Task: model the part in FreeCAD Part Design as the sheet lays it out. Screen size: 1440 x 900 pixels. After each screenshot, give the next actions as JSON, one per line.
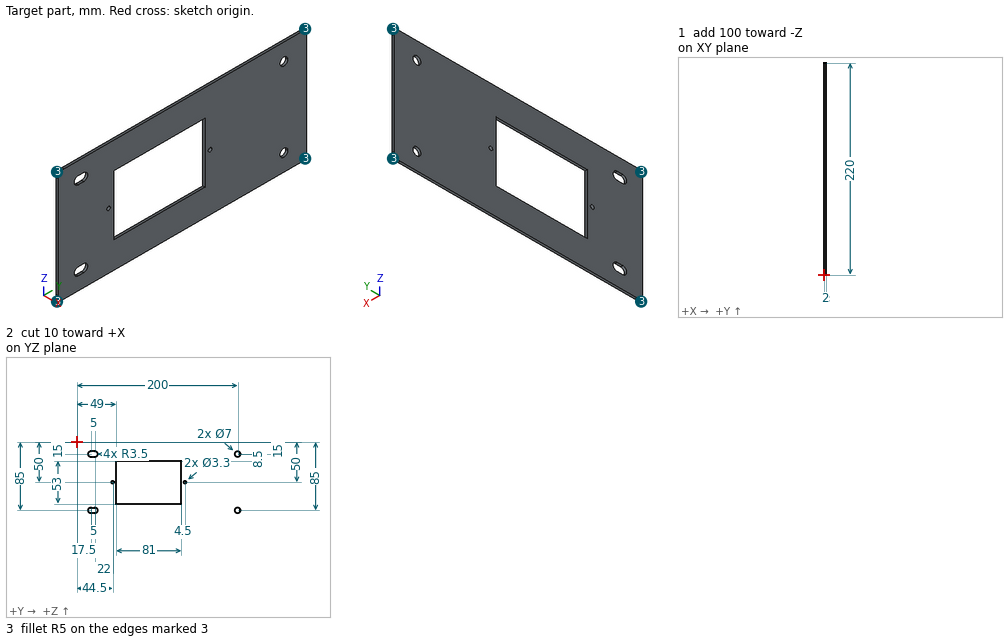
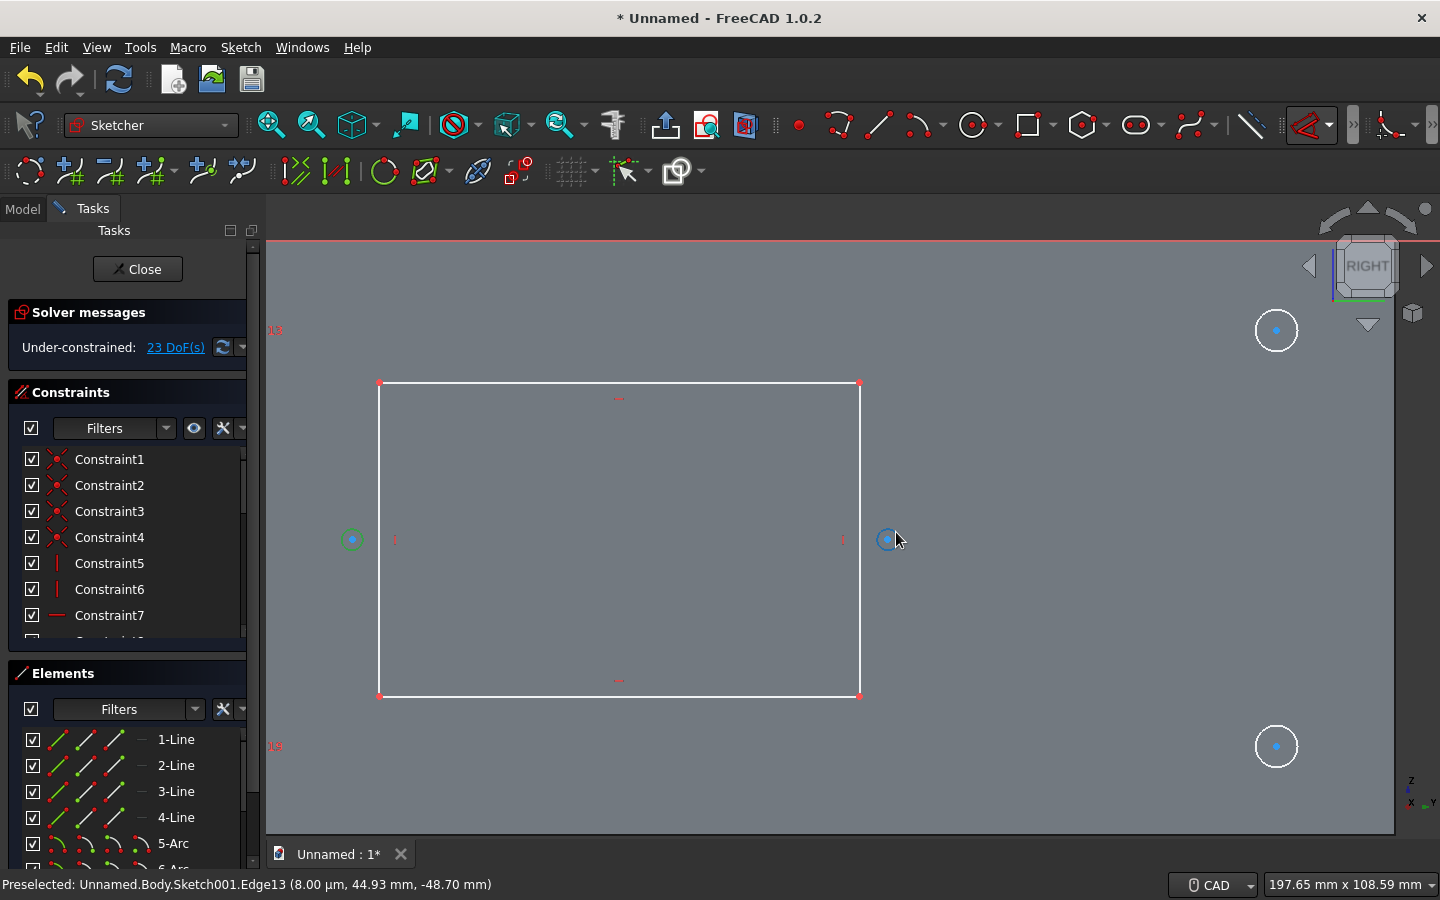
{"action": "left_click", "coordinate": [895, 532]}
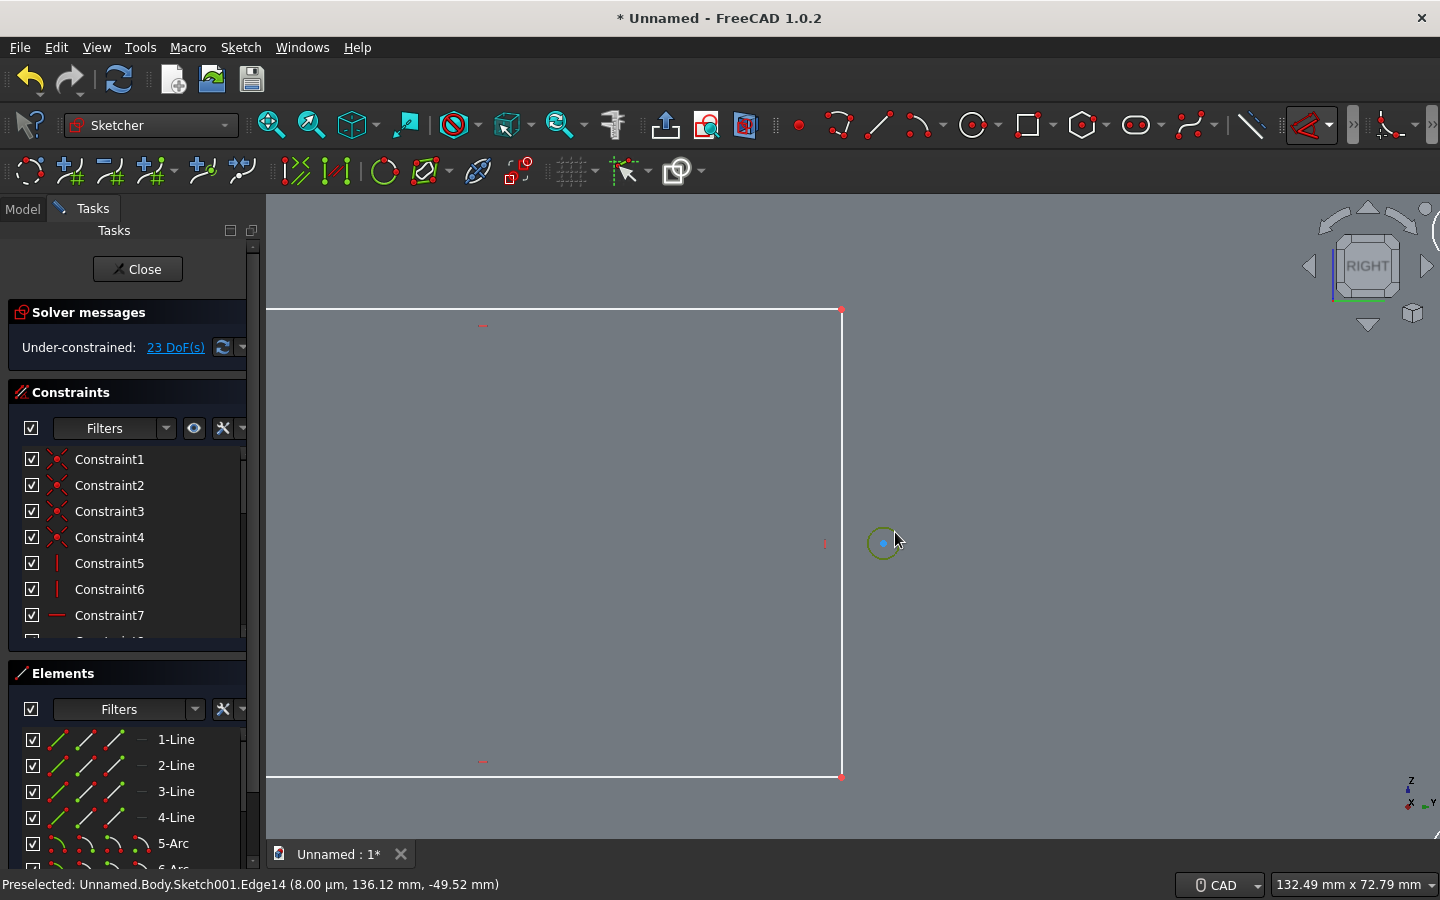
{"action": "key", "text": "e"}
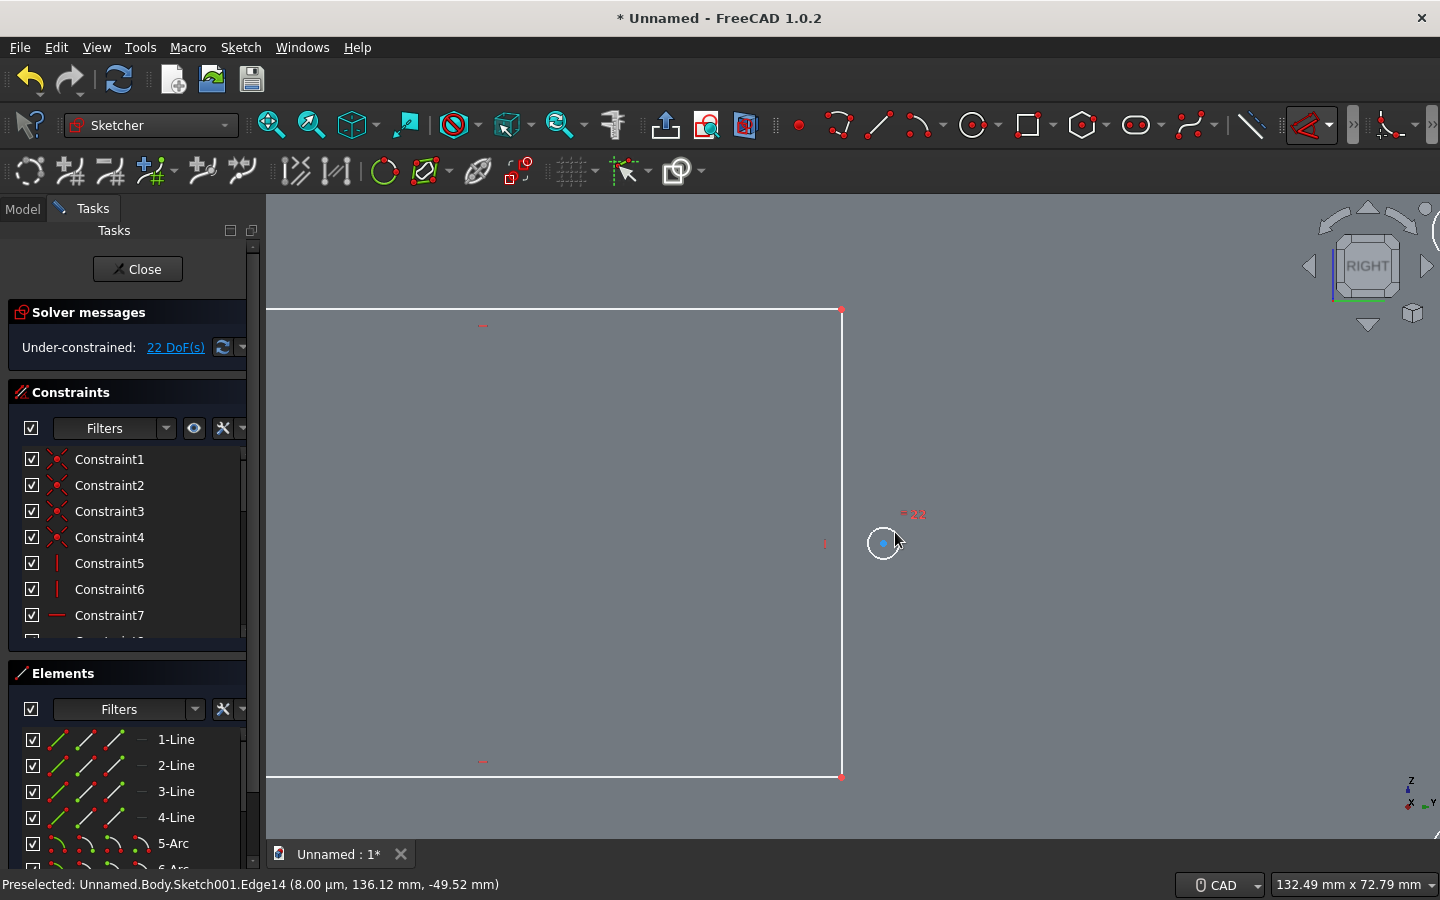
{"action": "scroll", "coordinate": [896, 532], "scroll_direction": "down", "scroll_amount": 5}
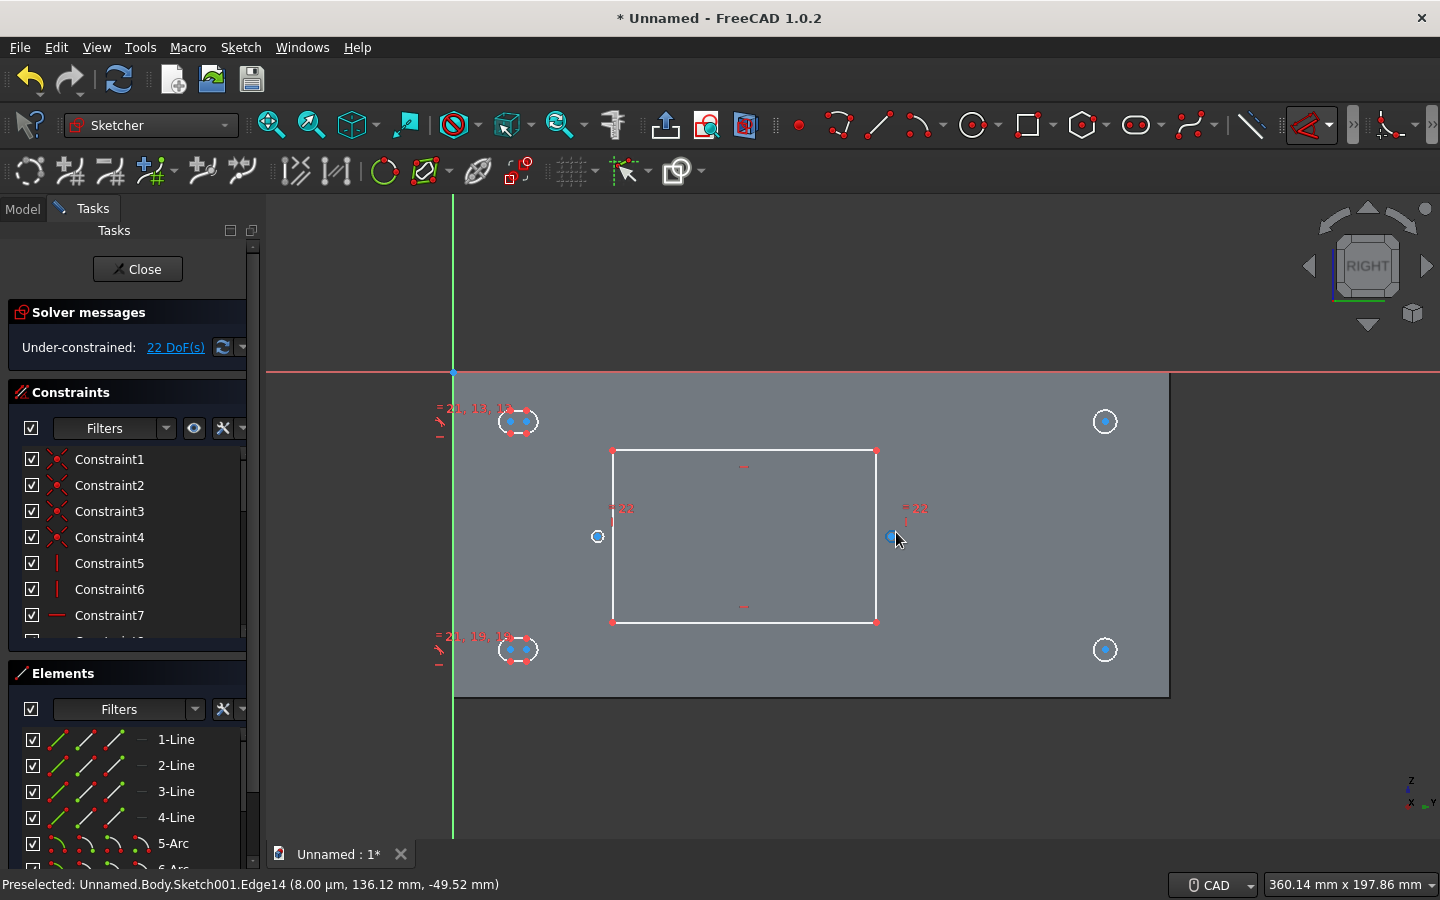
{"action": "left_click", "coordinate": [1113, 414]}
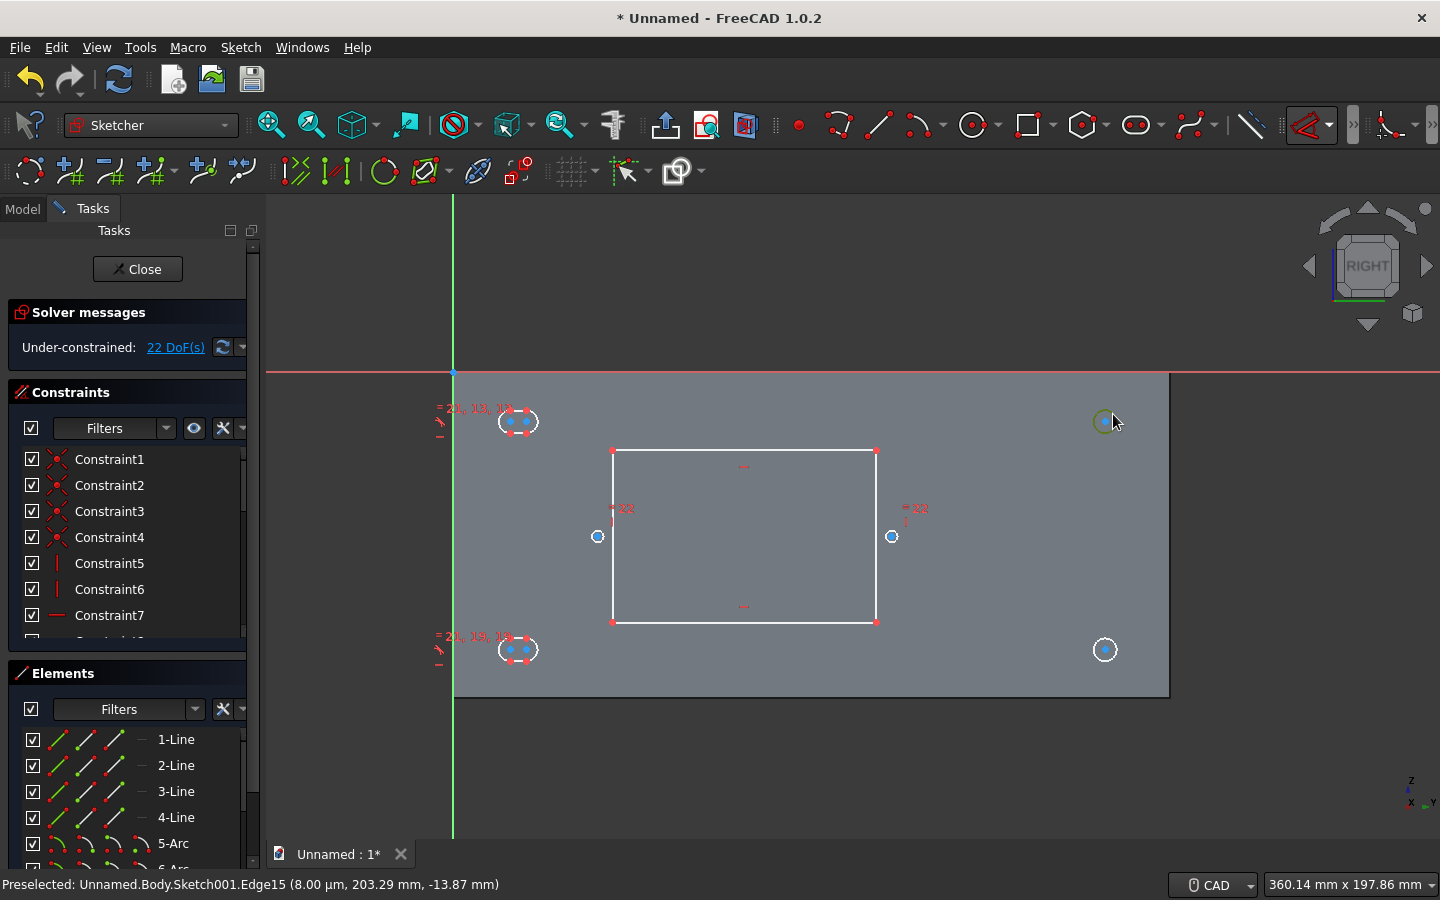
{"action": "left_click", "coordinate": [1113, 642]}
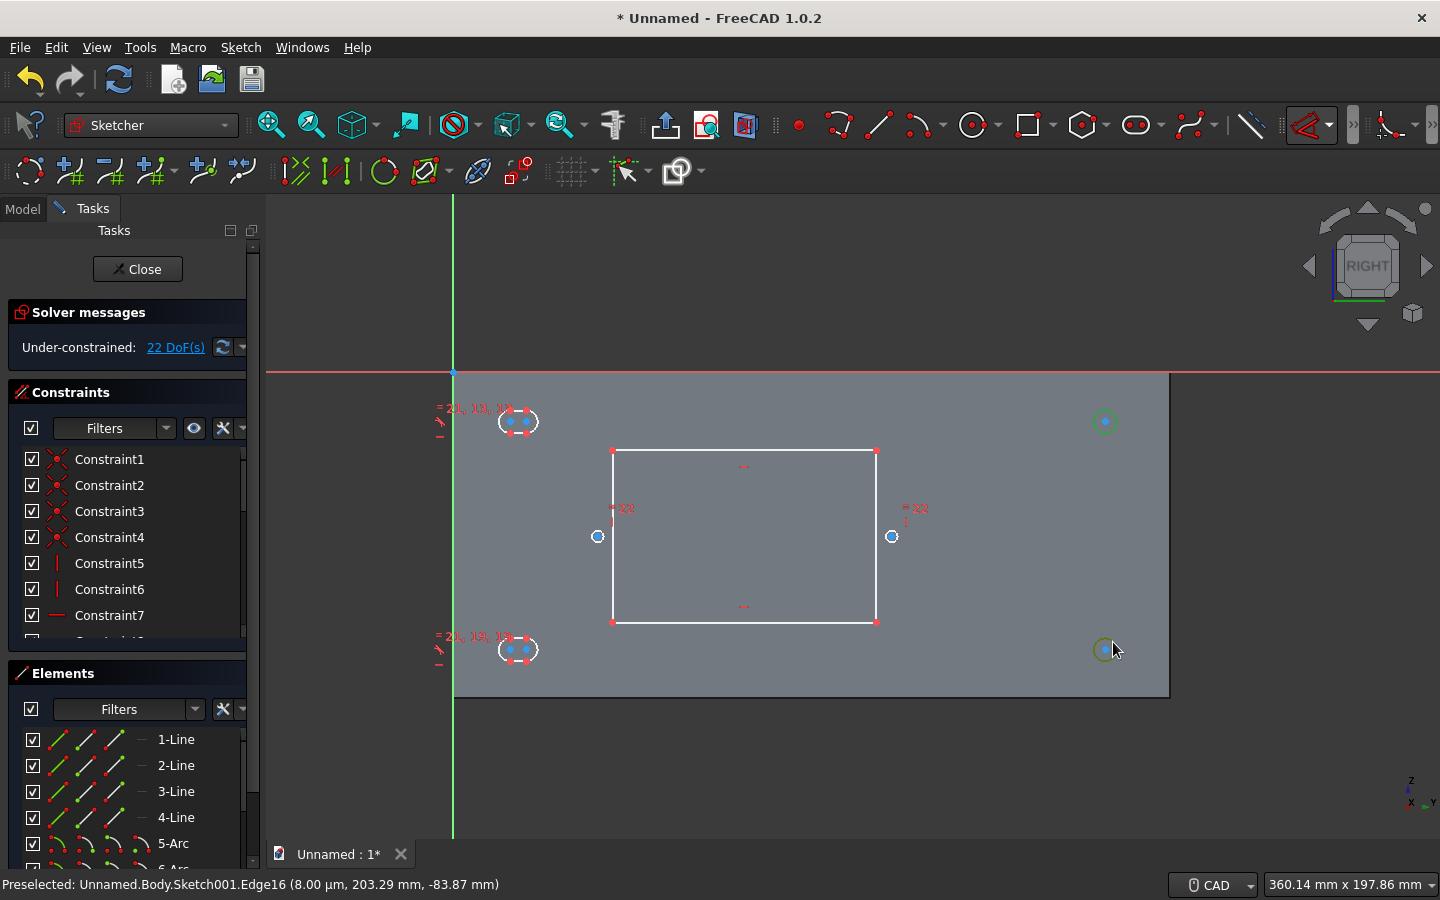
{"action": "key", "text": "e"}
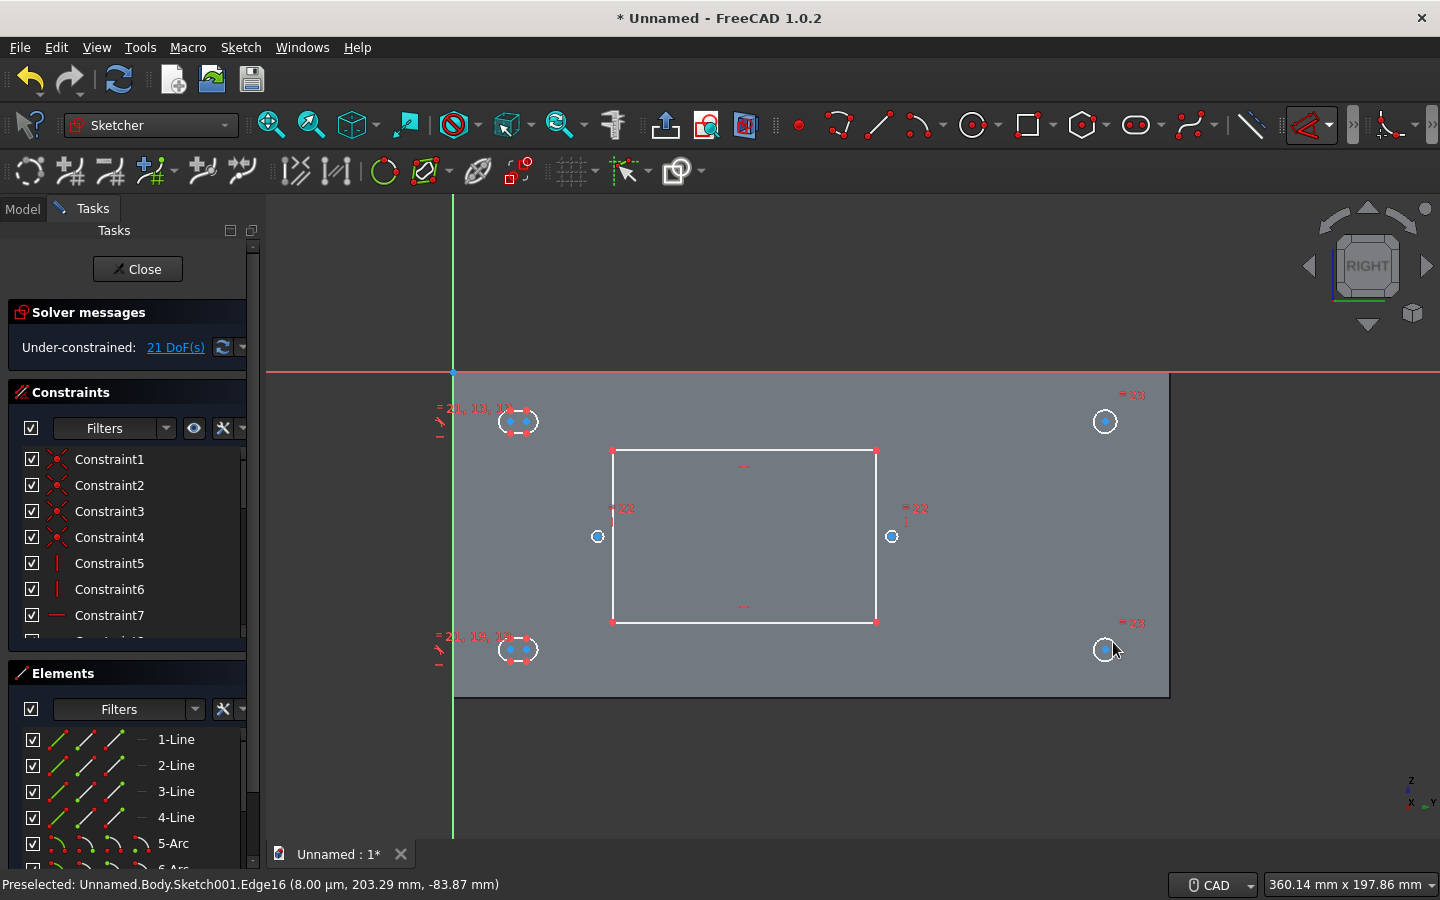
{"action": "left_click", "coordinate": [1105, 422]}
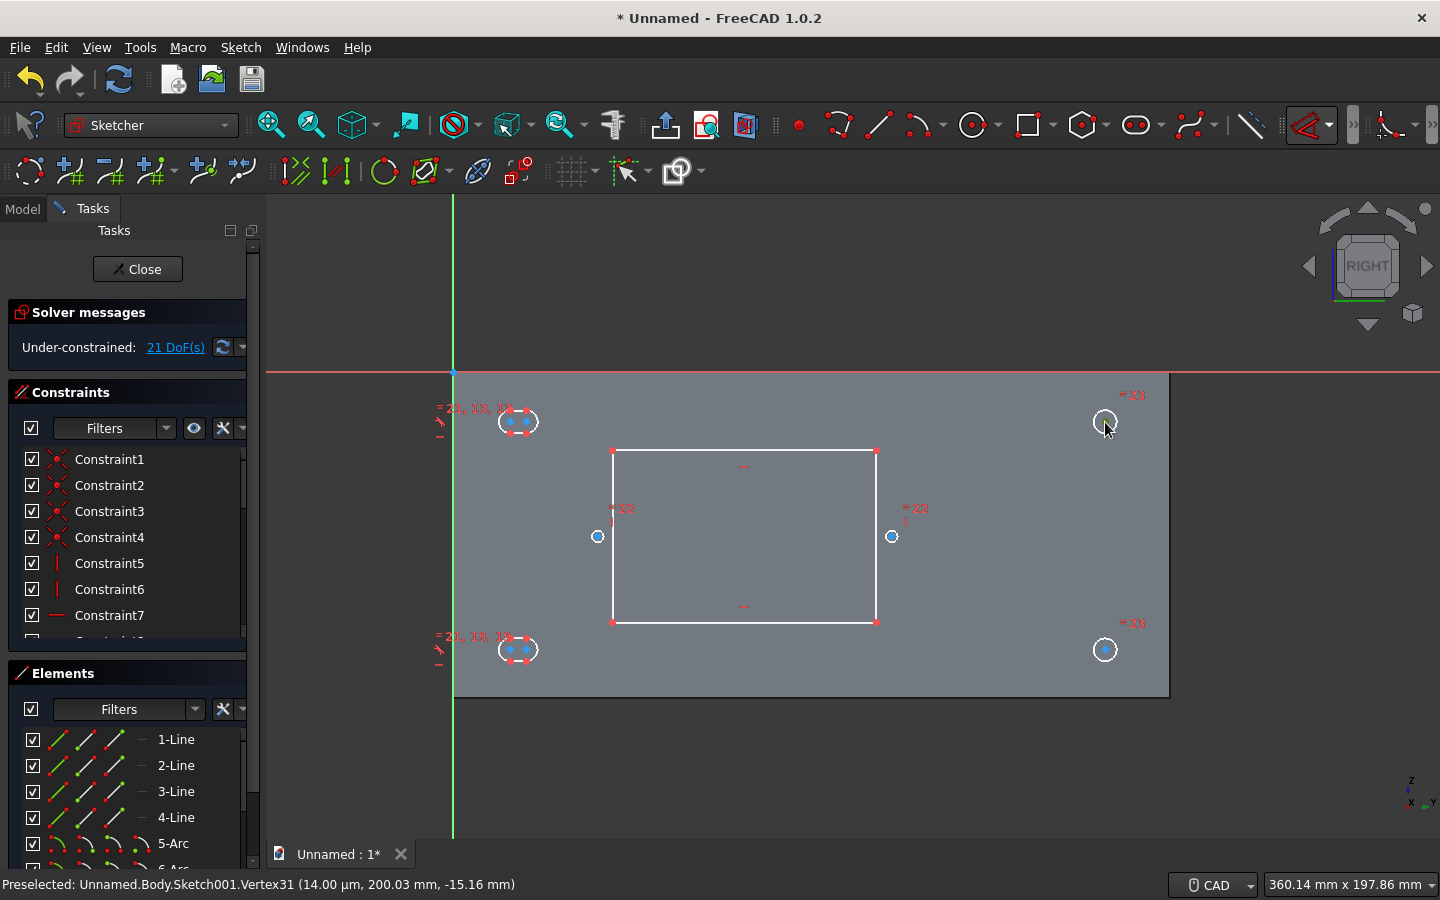
{"action": "left_click", "coordinate": [1105, 650]}